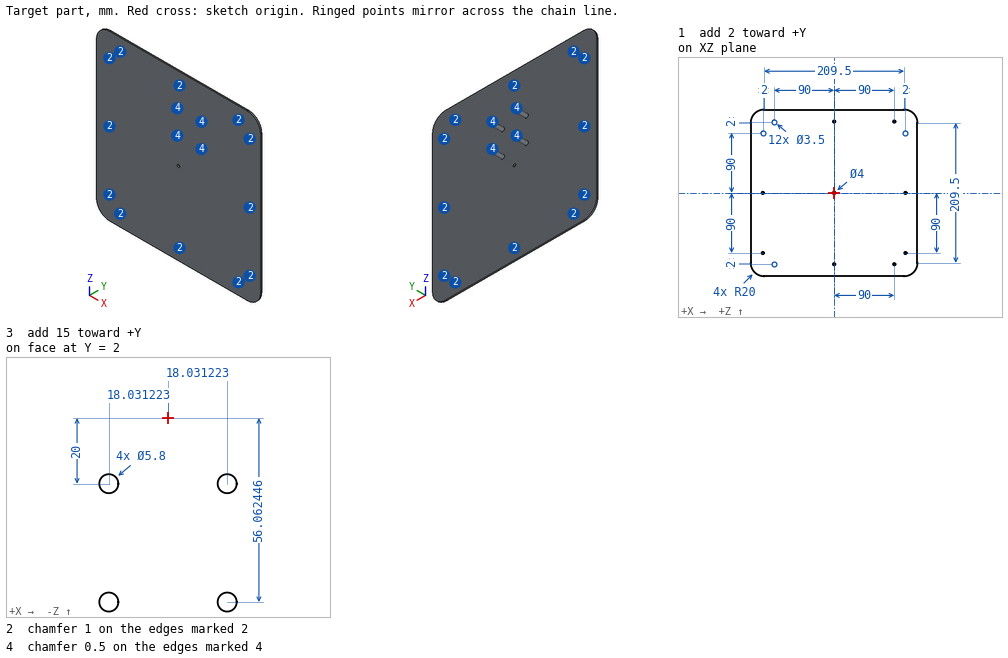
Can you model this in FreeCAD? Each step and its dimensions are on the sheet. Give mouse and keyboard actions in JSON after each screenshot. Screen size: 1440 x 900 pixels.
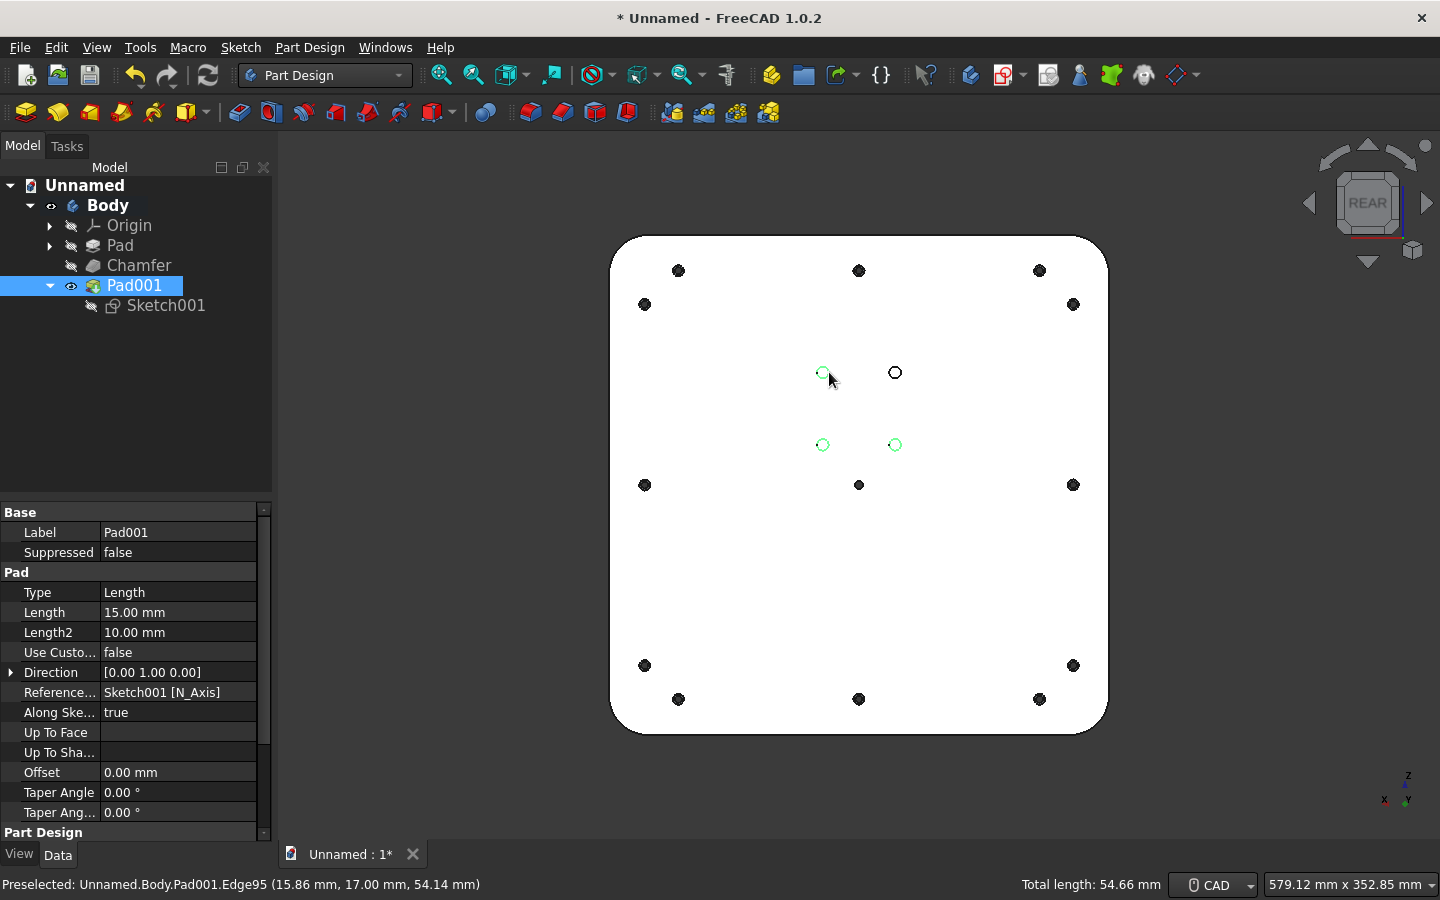
{"action": "left_click", "coordinate": [901, 372], "text": "ctrl"}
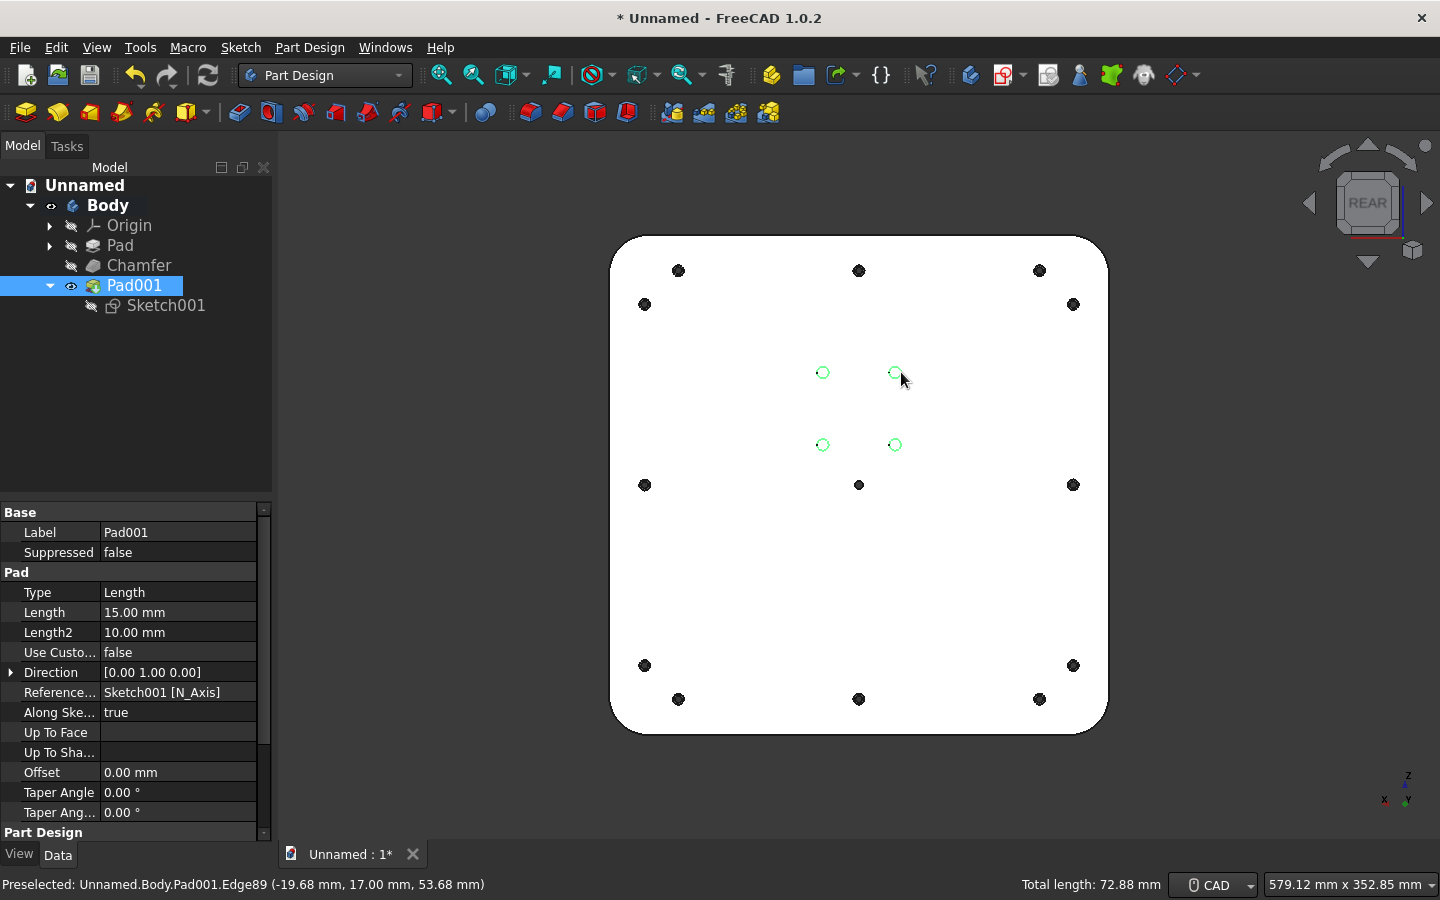
{"action": "left_click", "coordinate": [564, 112]}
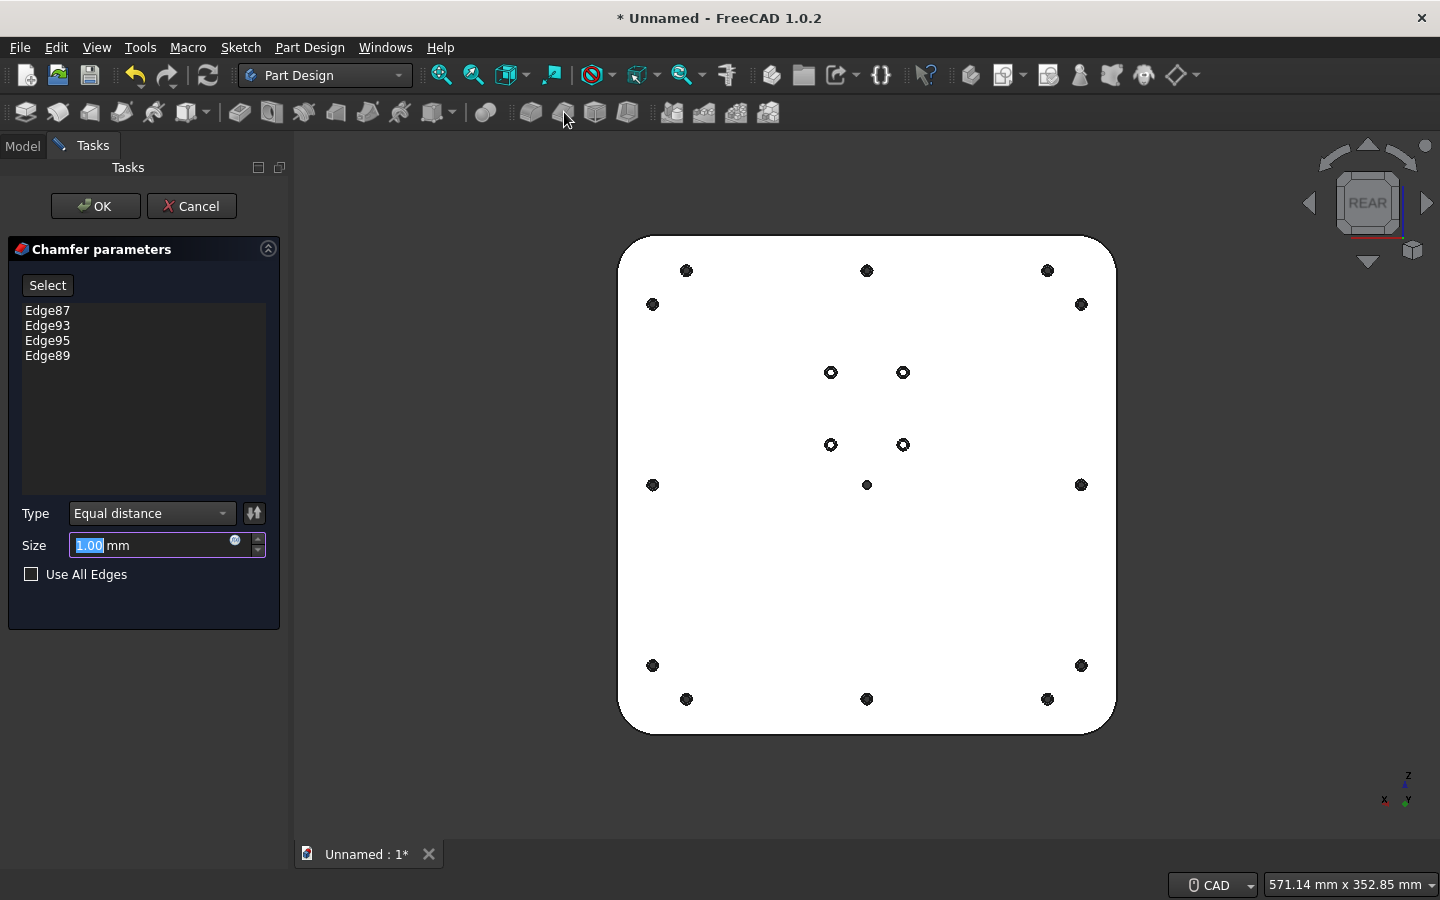
{"action": "type", "text": "0.5"}
{"action": "key", "text": "Tab"}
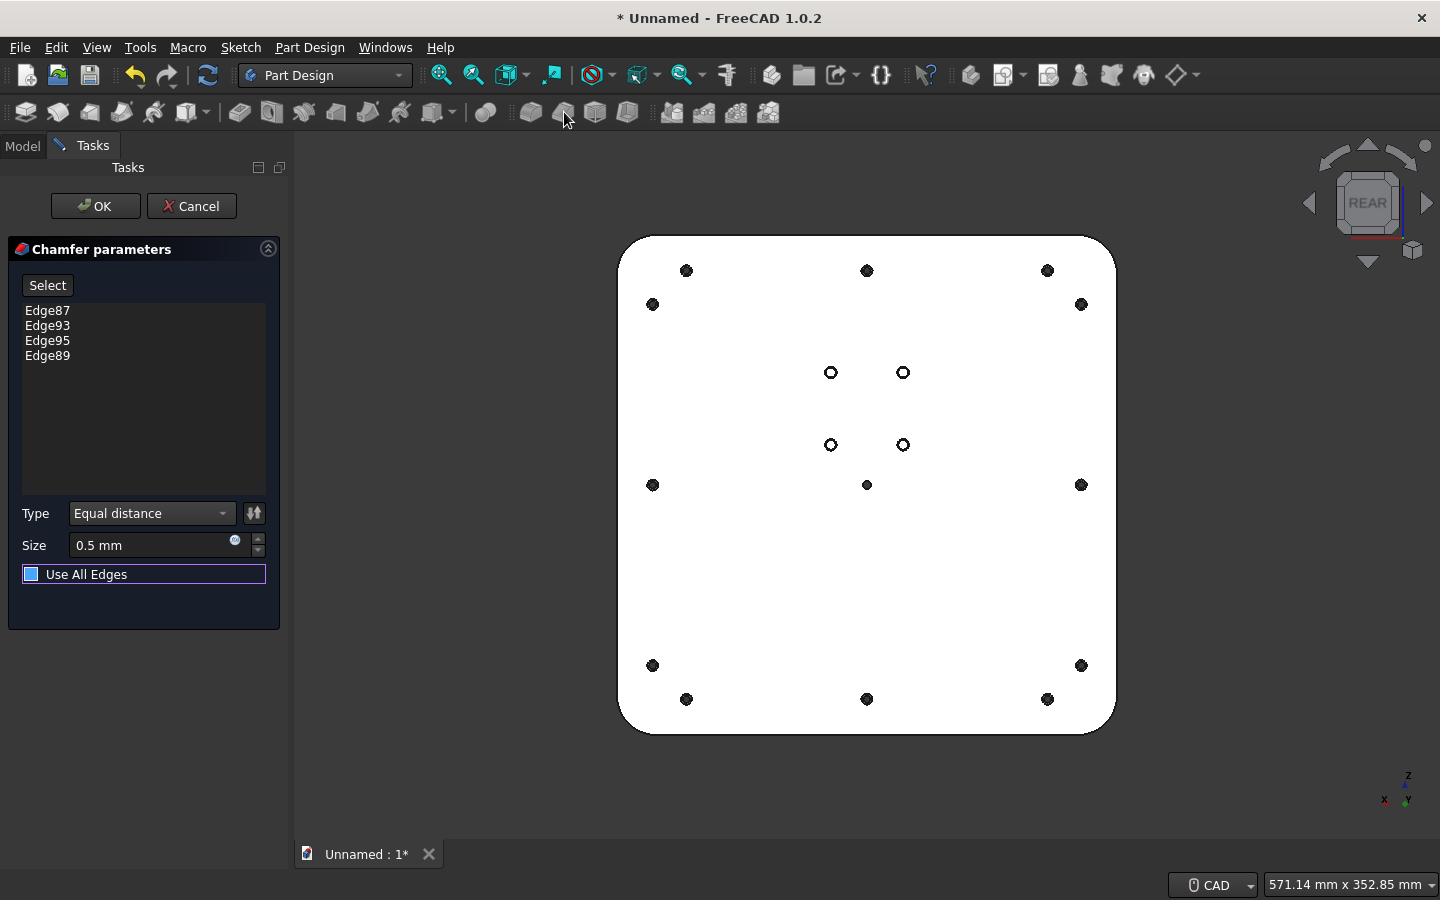
{"action": "left_click", "coordinate": [96, 206]}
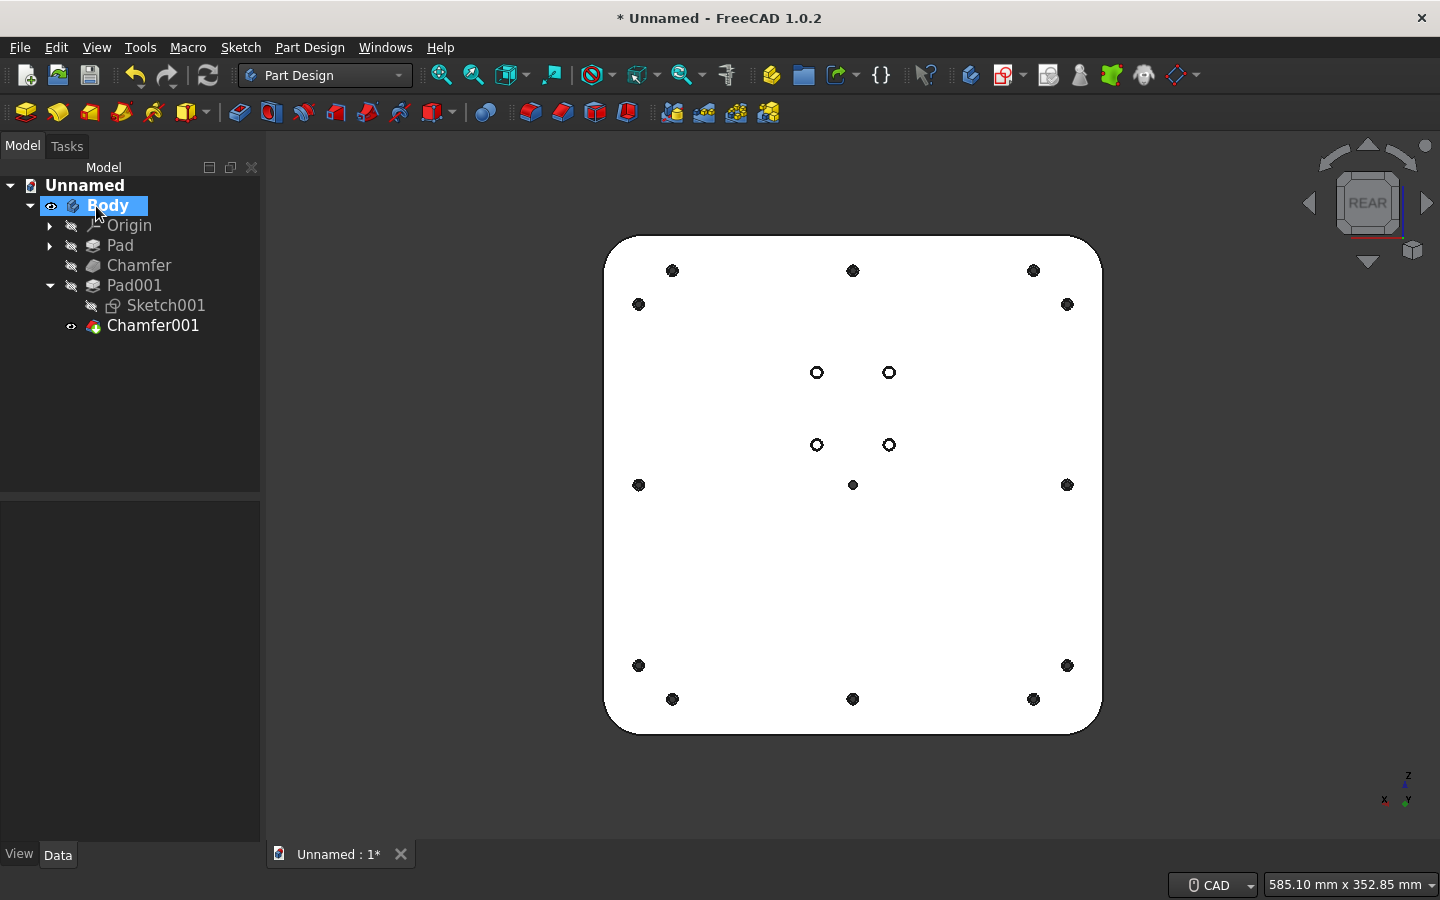
{"action": "key", "text": "0"}